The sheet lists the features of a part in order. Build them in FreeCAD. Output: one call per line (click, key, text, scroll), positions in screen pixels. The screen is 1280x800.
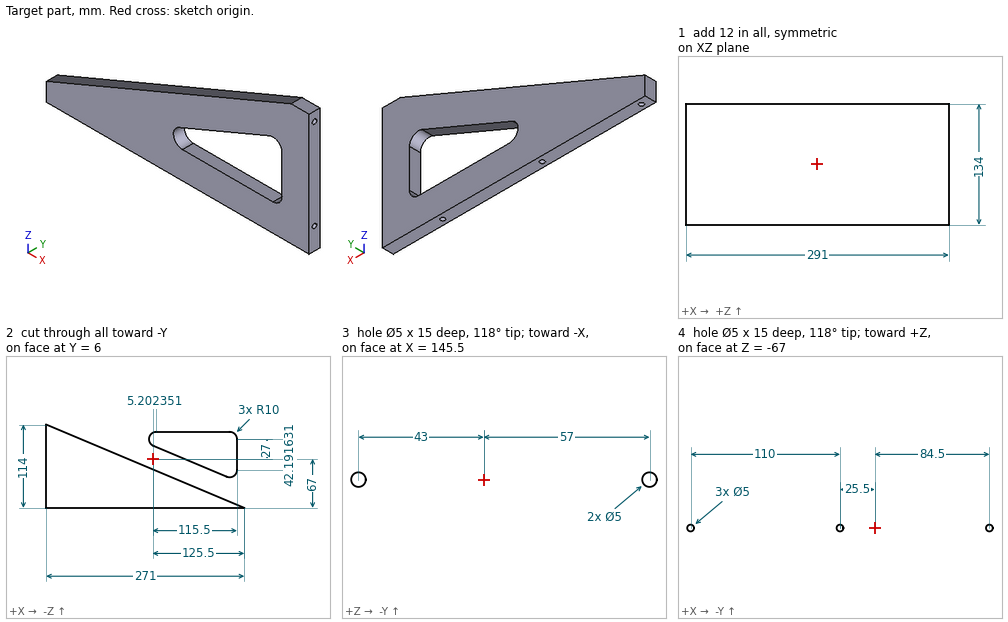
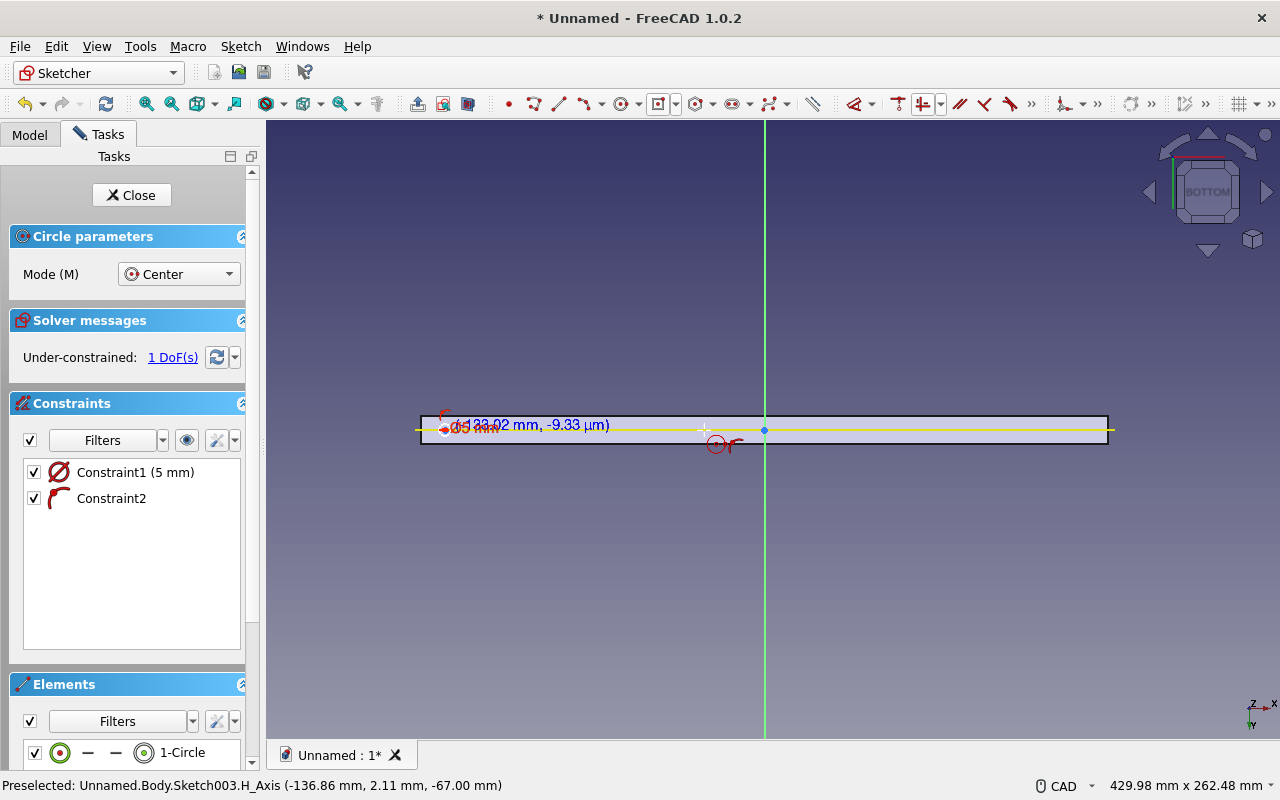
click(704, 430)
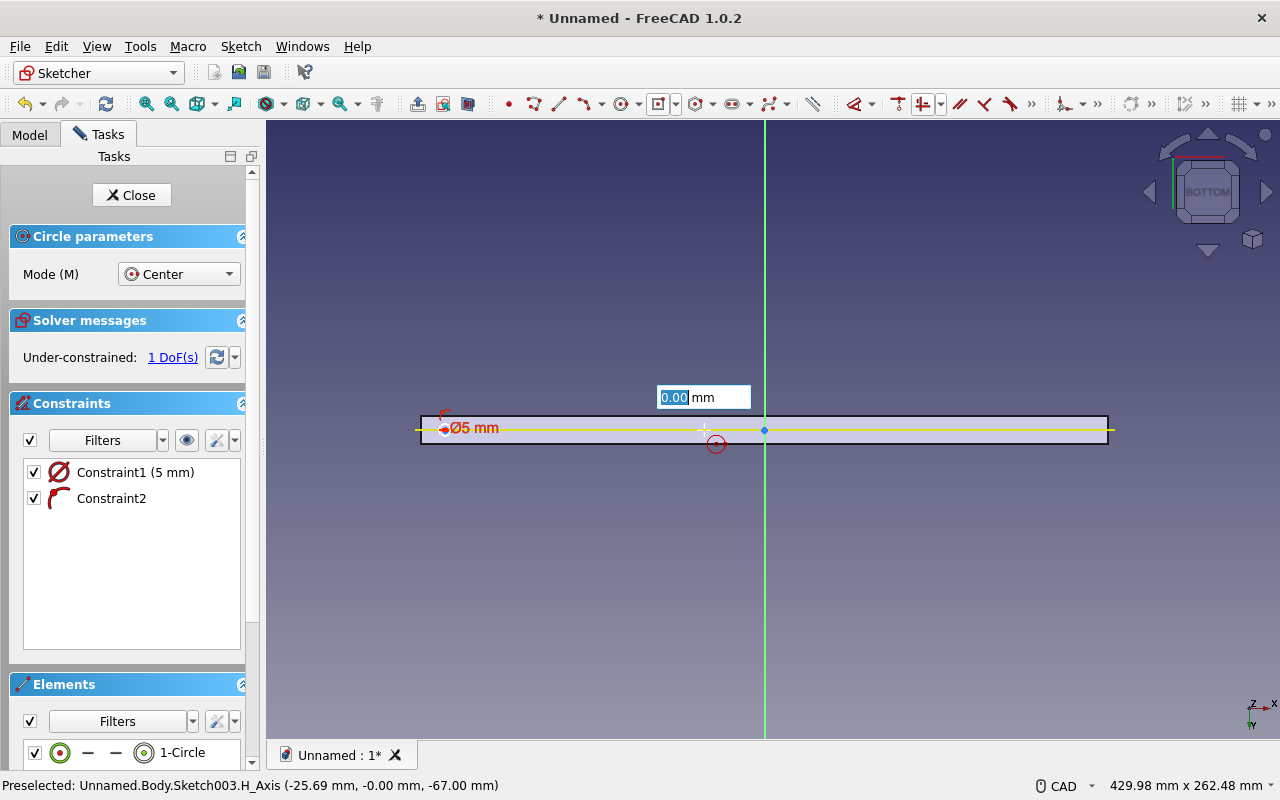
scroll(702, 436, up, 6)
move(702, 433)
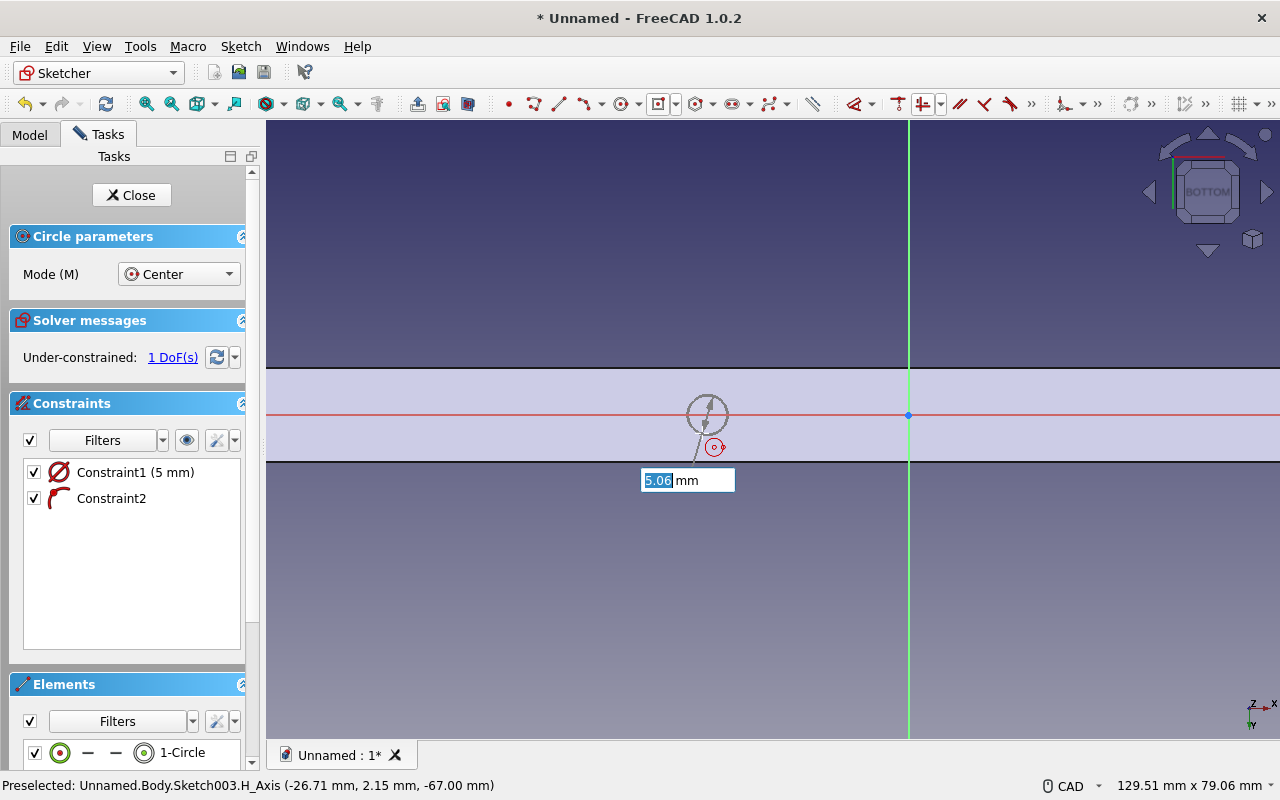
text(5)
key(Return)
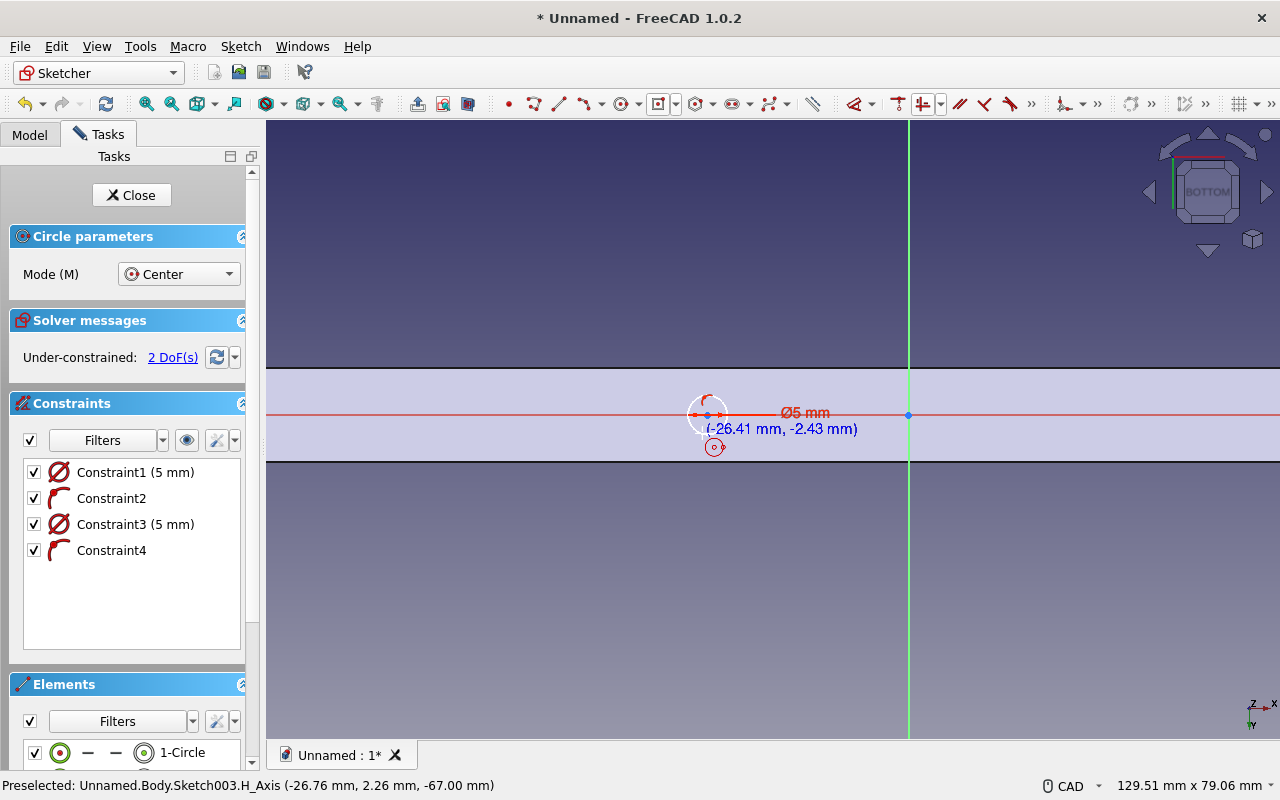
scroll(702, 436, down, 6)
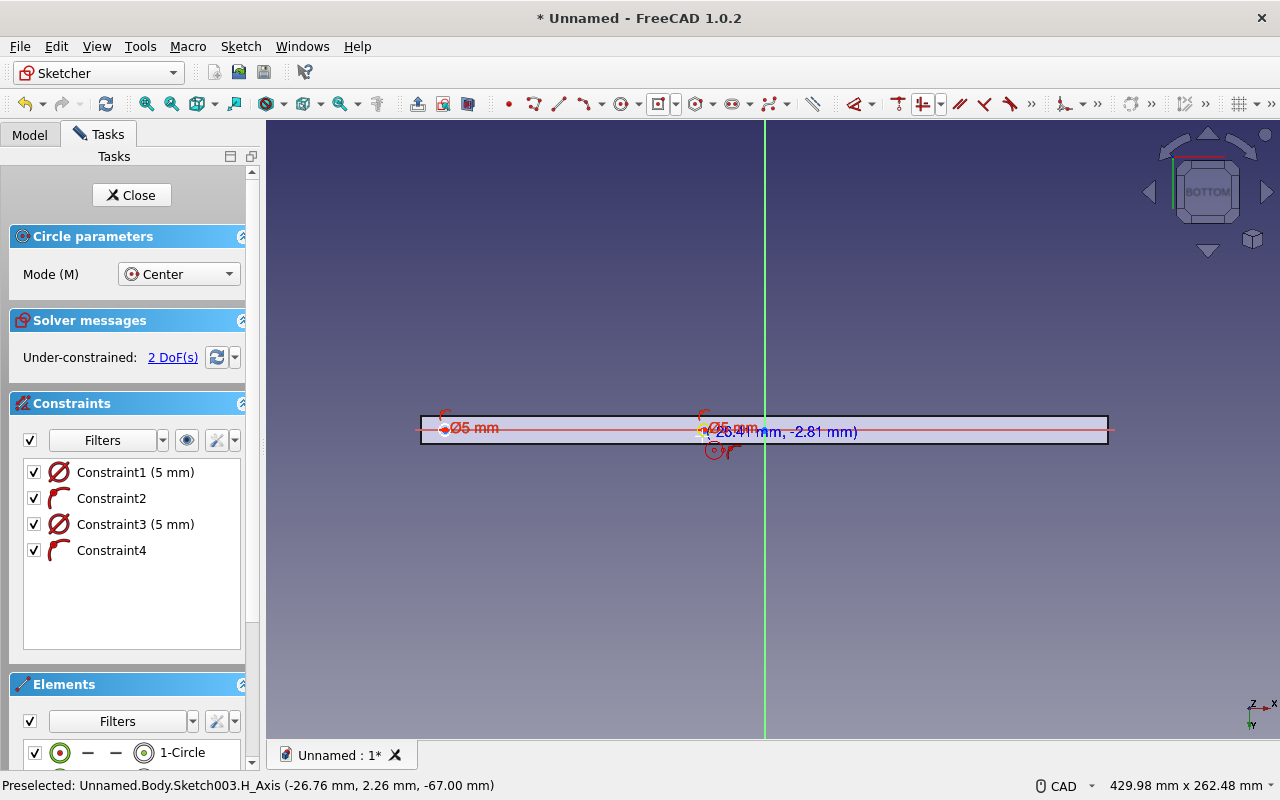
scroll(964, 430, up, 7)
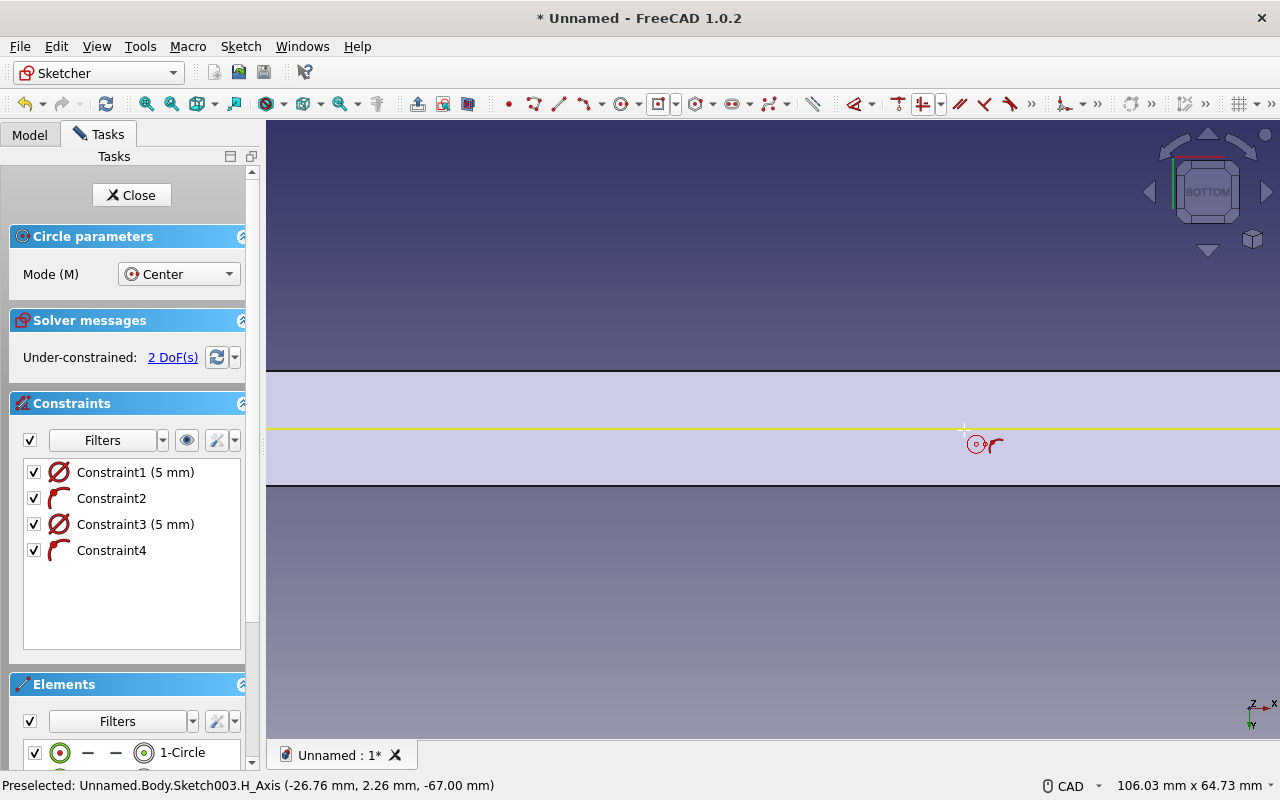
scroll(965, 430, down, 7)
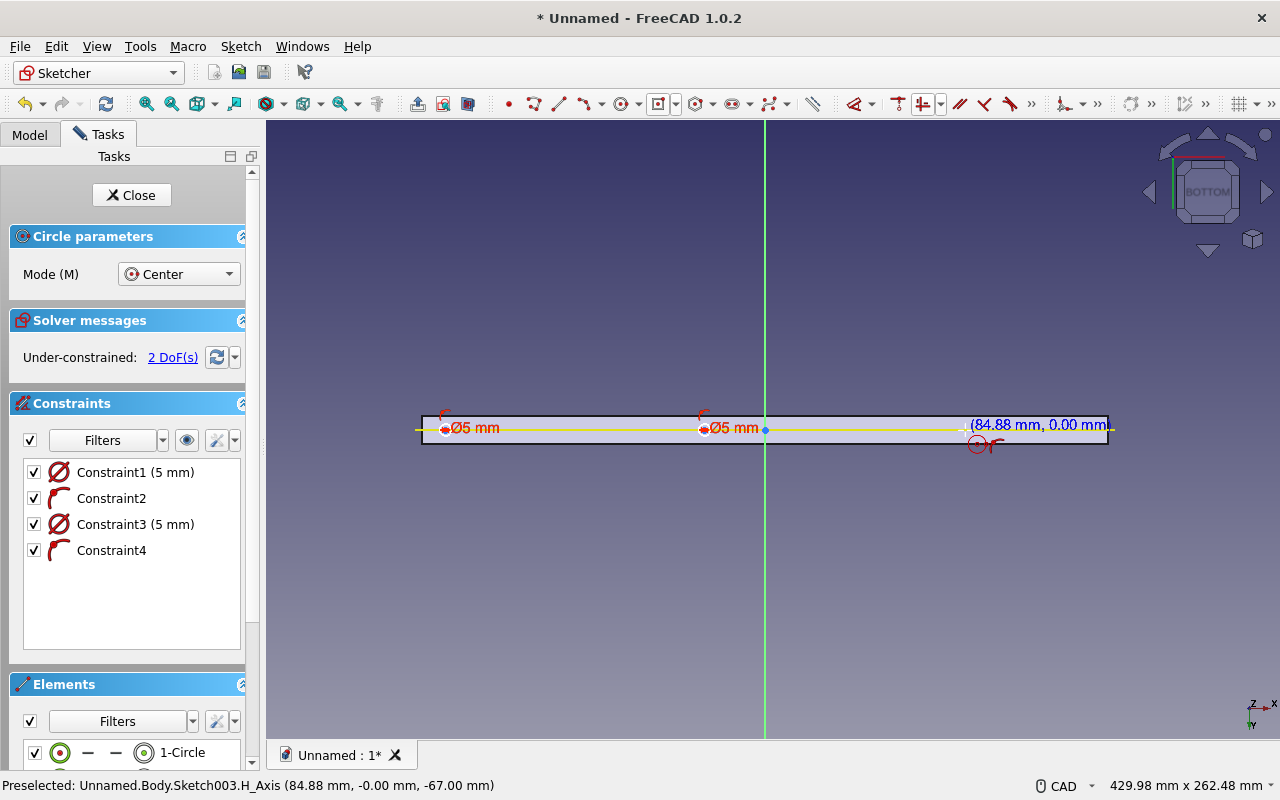
click(965, 430)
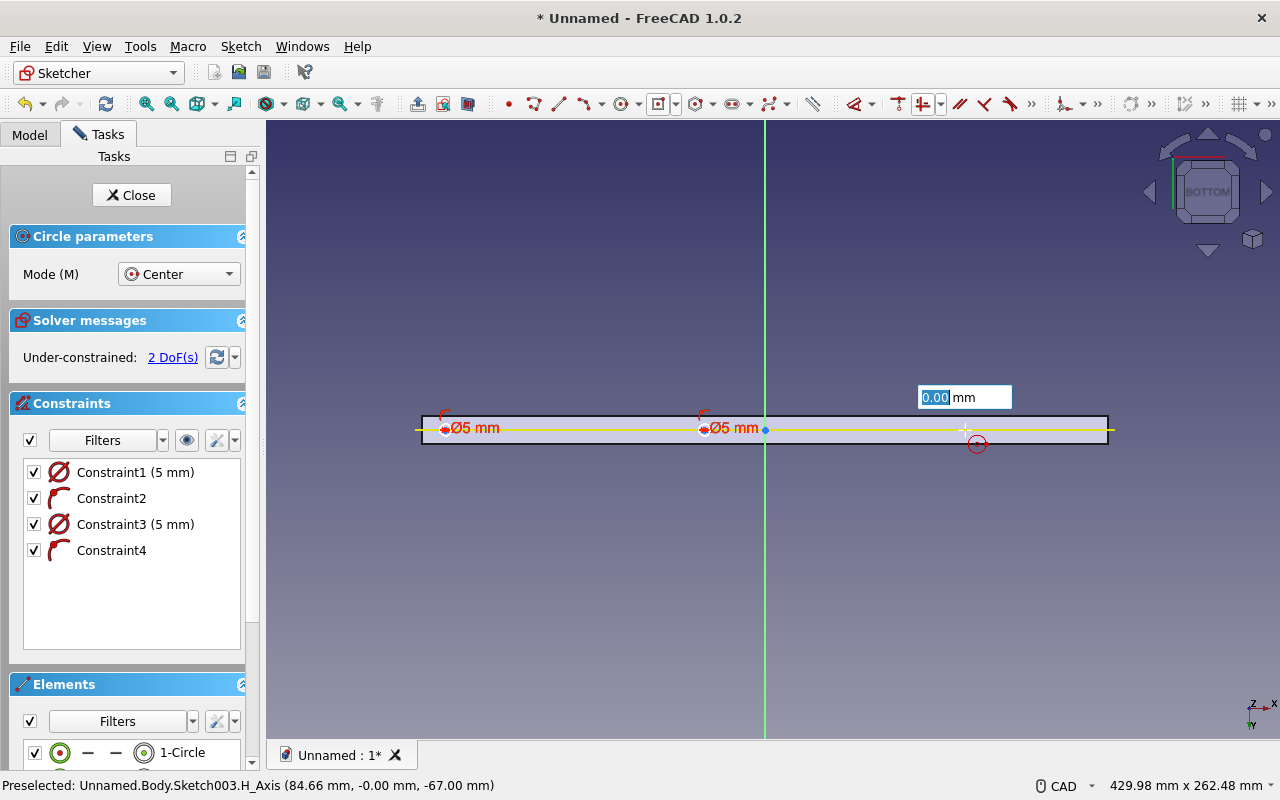
scroll(963, 436, up, 6)
move(960, 433)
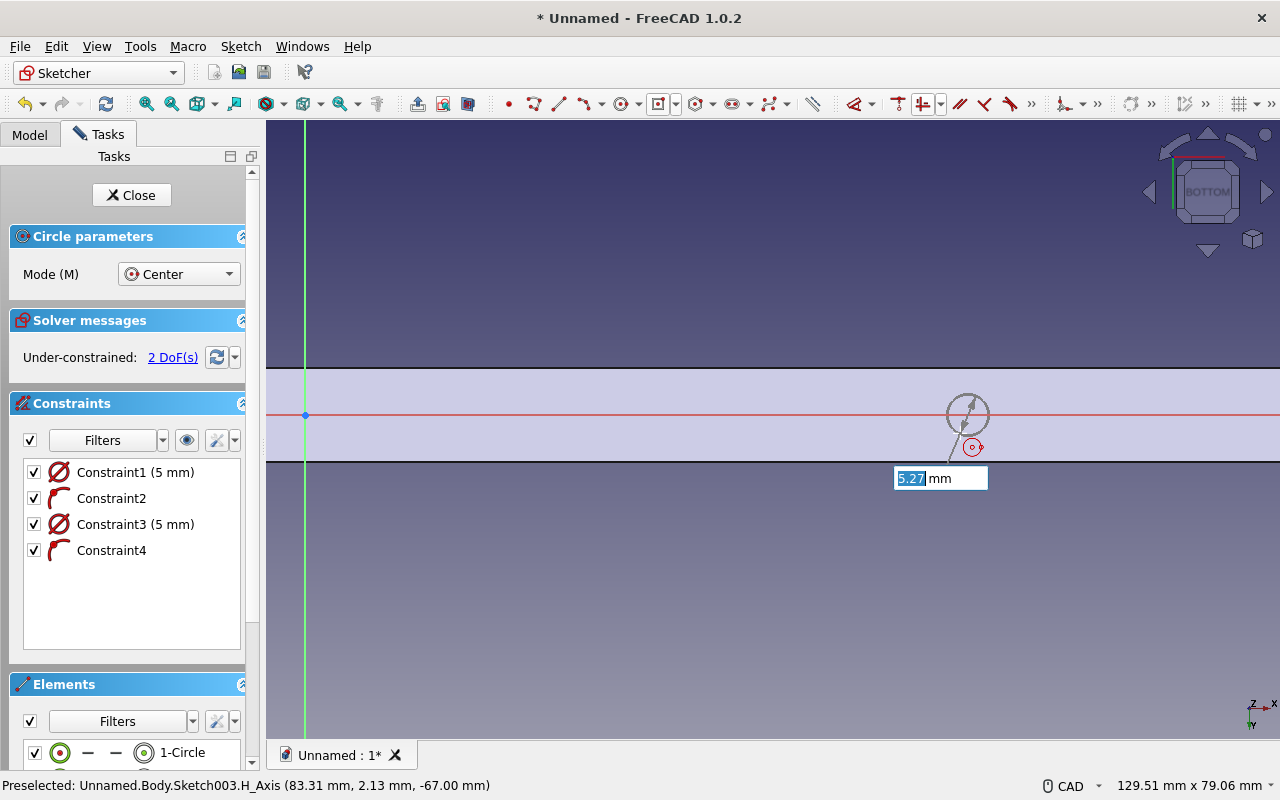
text(5)
key(Return)
key(Escape)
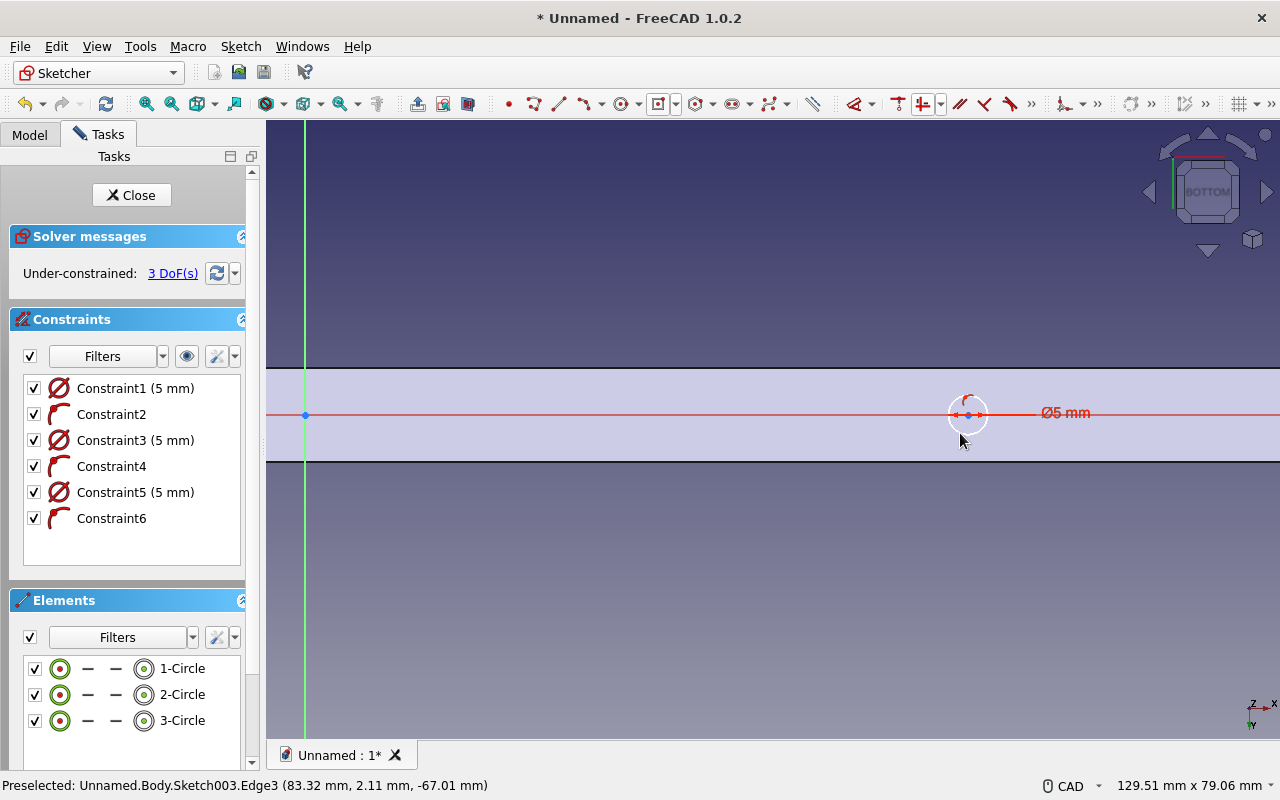
click(854, 104)